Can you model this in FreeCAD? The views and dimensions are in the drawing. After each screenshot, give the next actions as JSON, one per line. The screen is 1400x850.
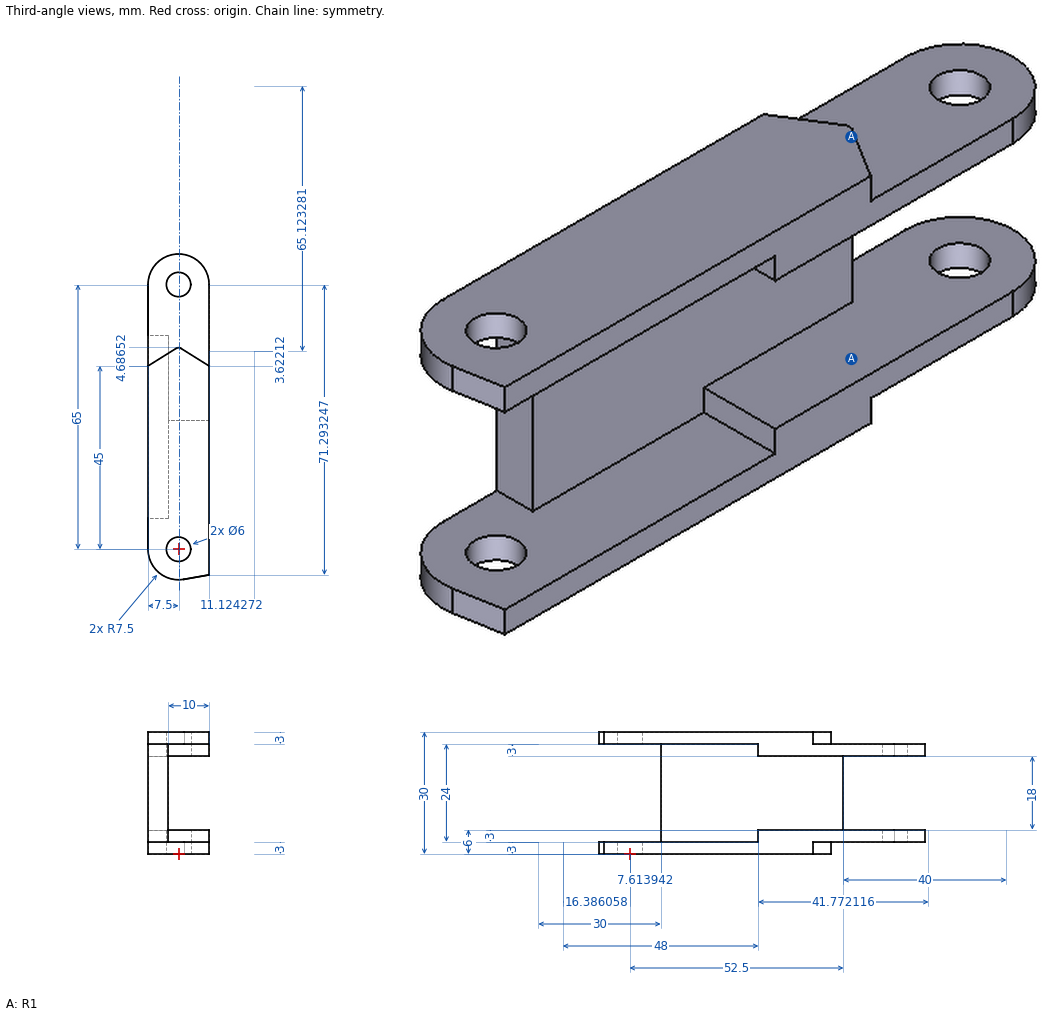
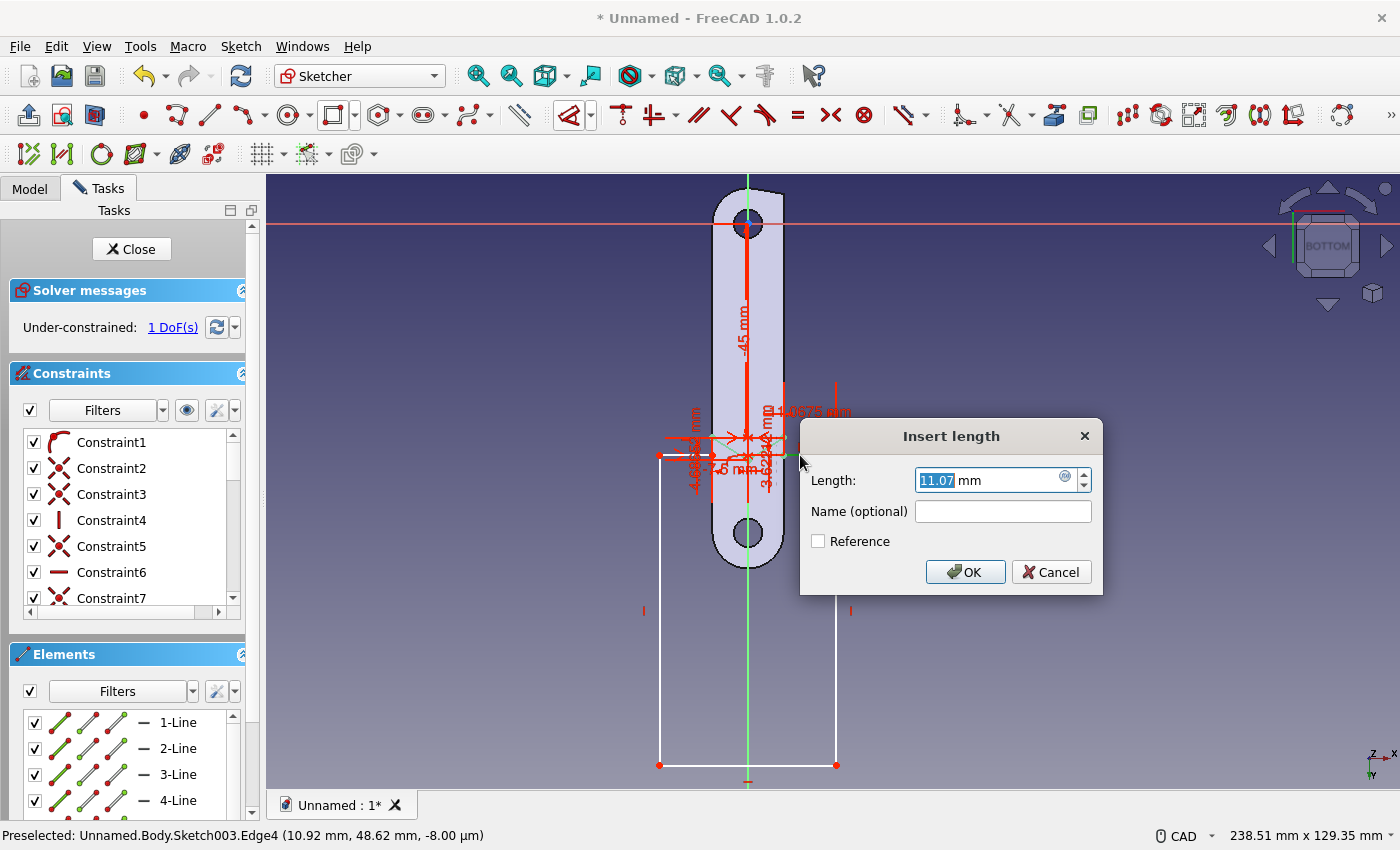
{"action": "type", "text": "11.124272"}
{"action": "key", "text": "Return"}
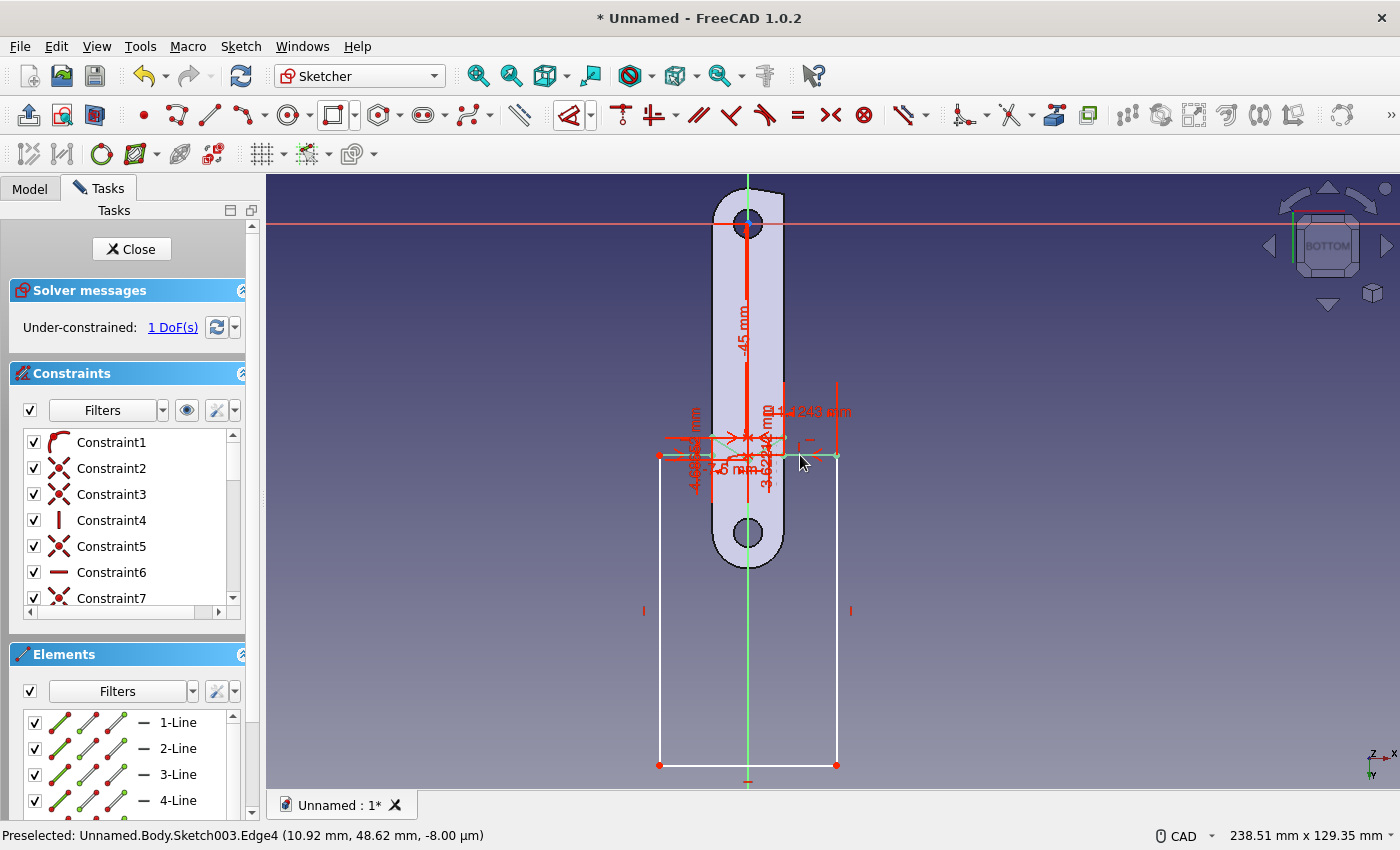
{"action": "left_click", "coordinate": [837, 548]}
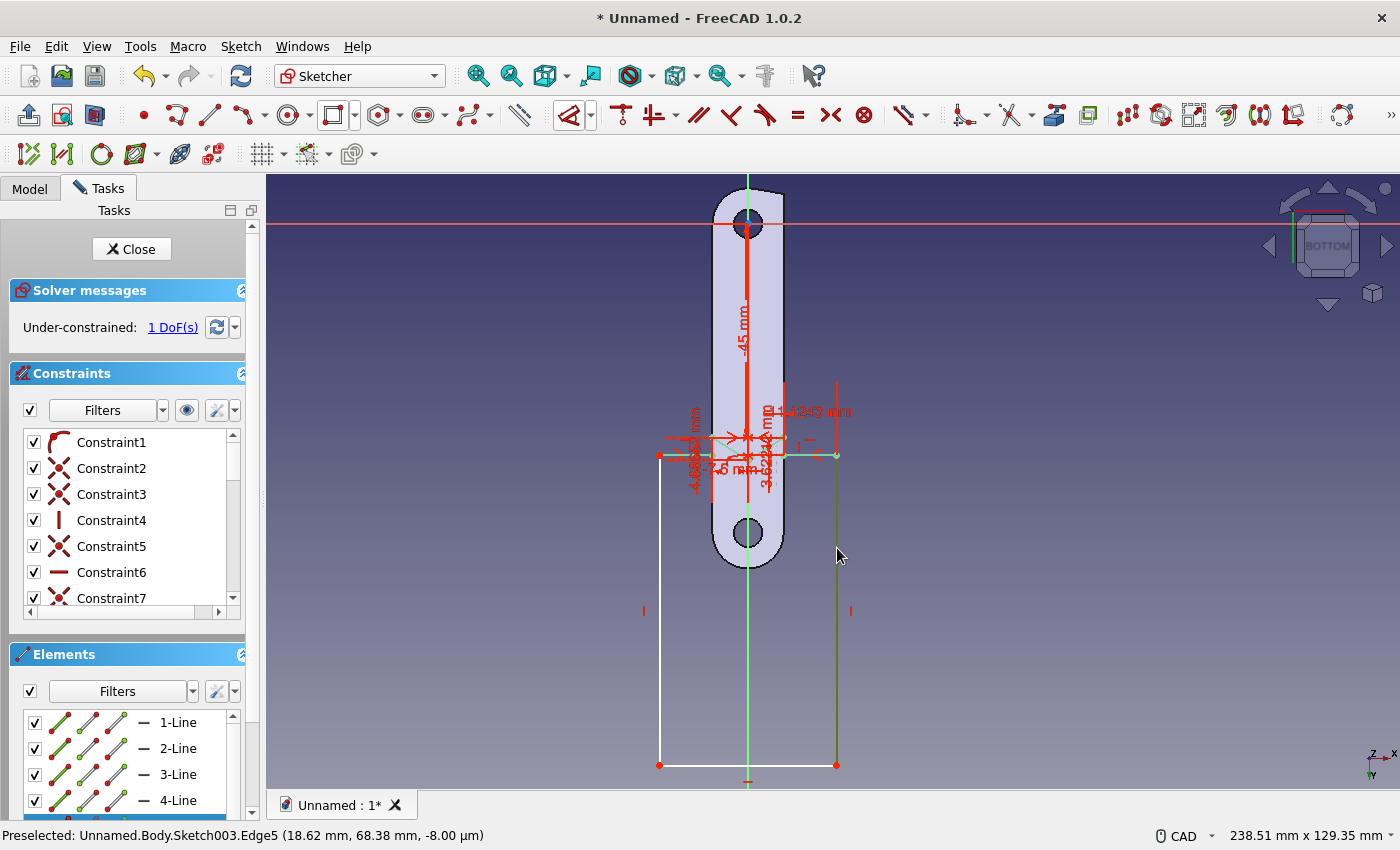
{"action": "key", "text": "i"}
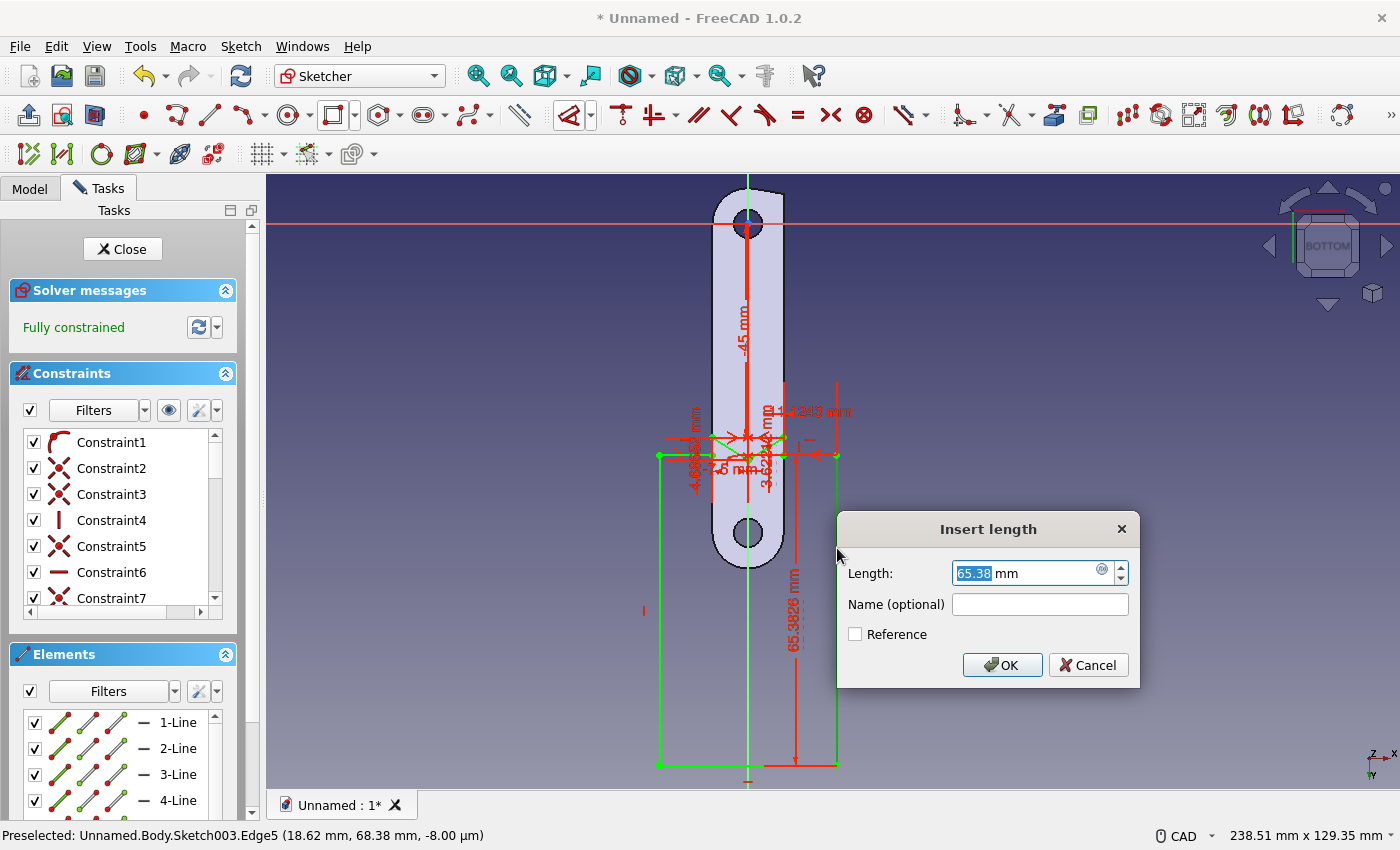
{"action": "type", "text": "65.123281"}
{"action": "key", "text": "Return"}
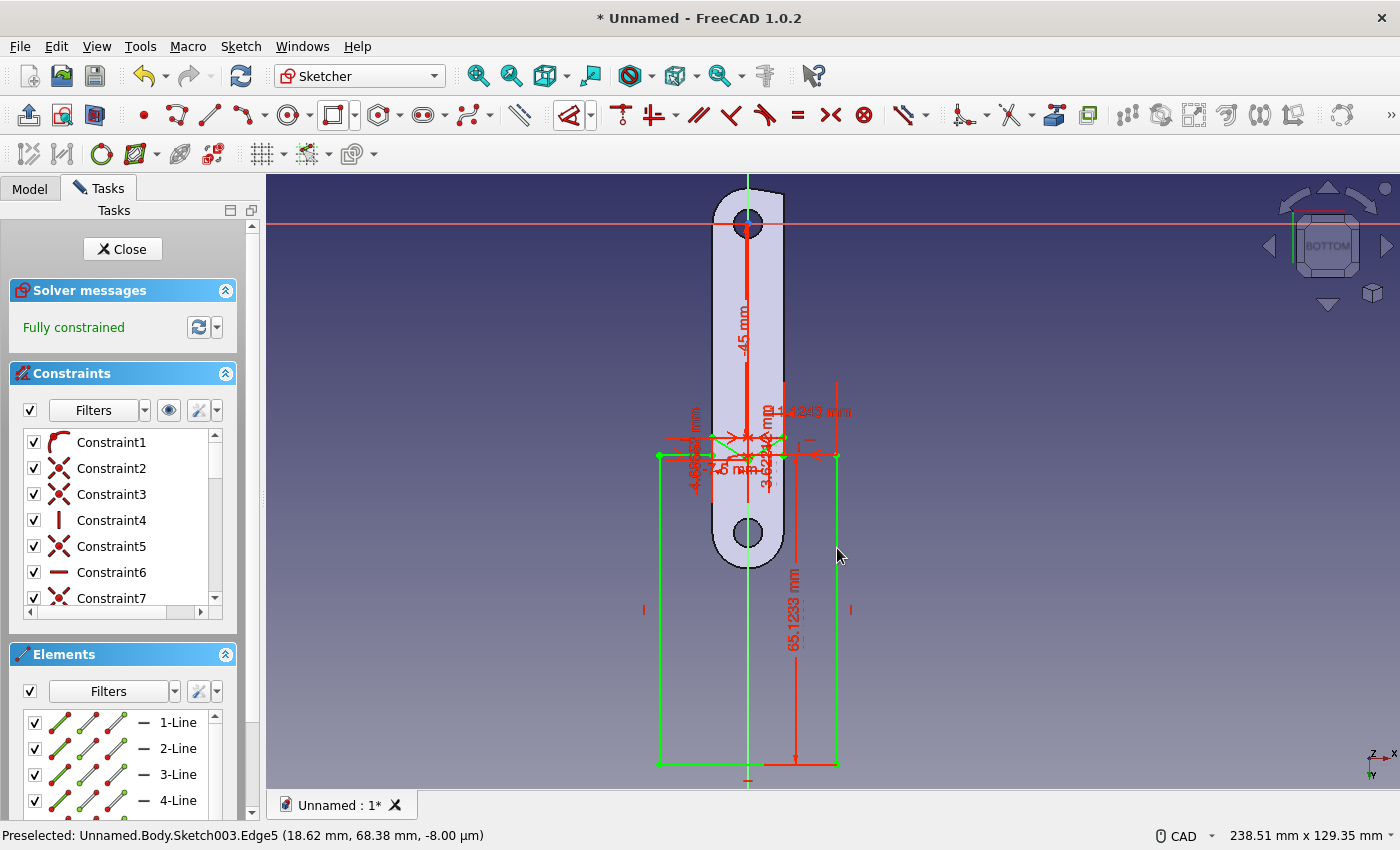
{"action": "left_click", "coordinate": [123, 249]}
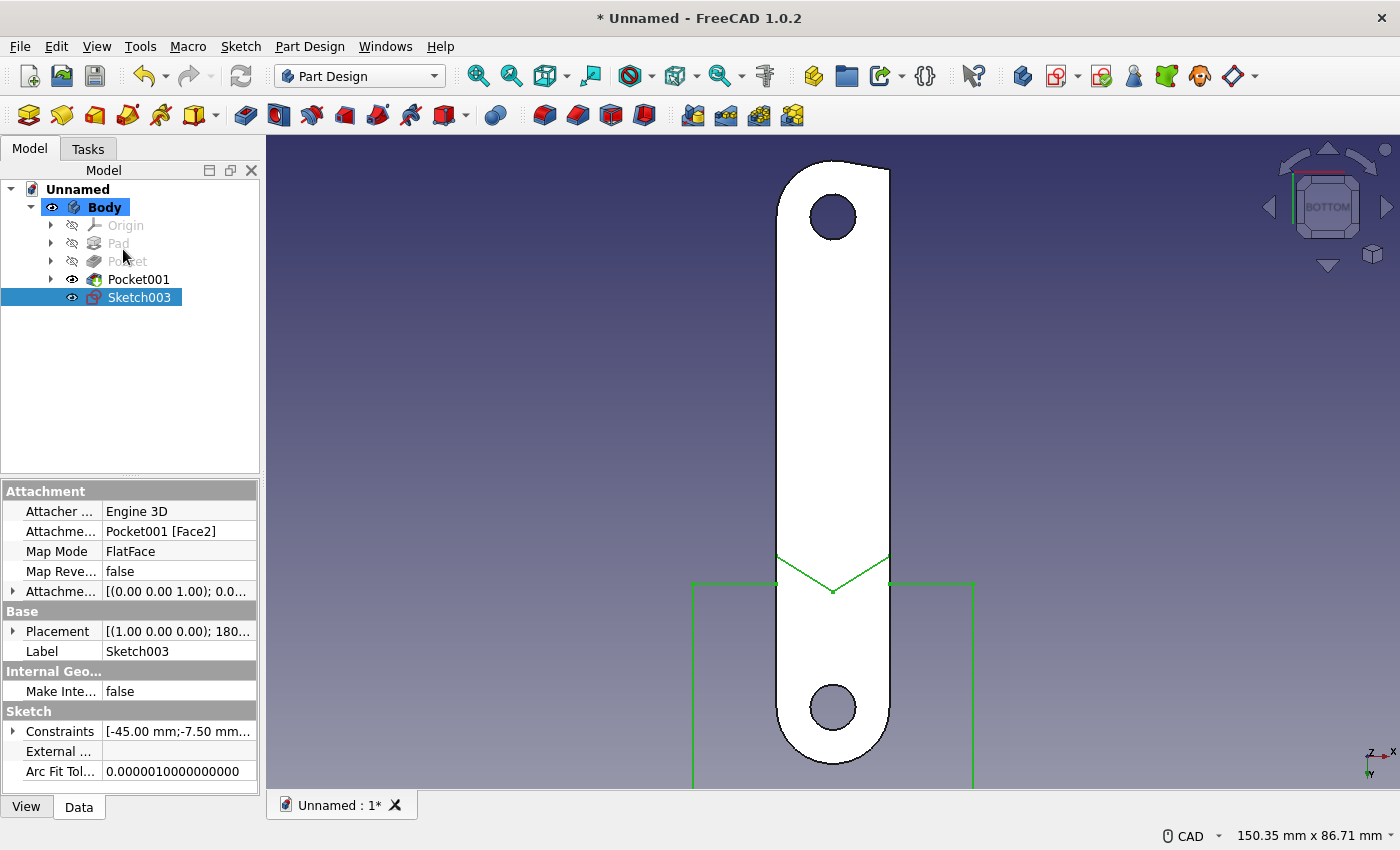
{"action": "left_click", "coordinate": [246, 116]}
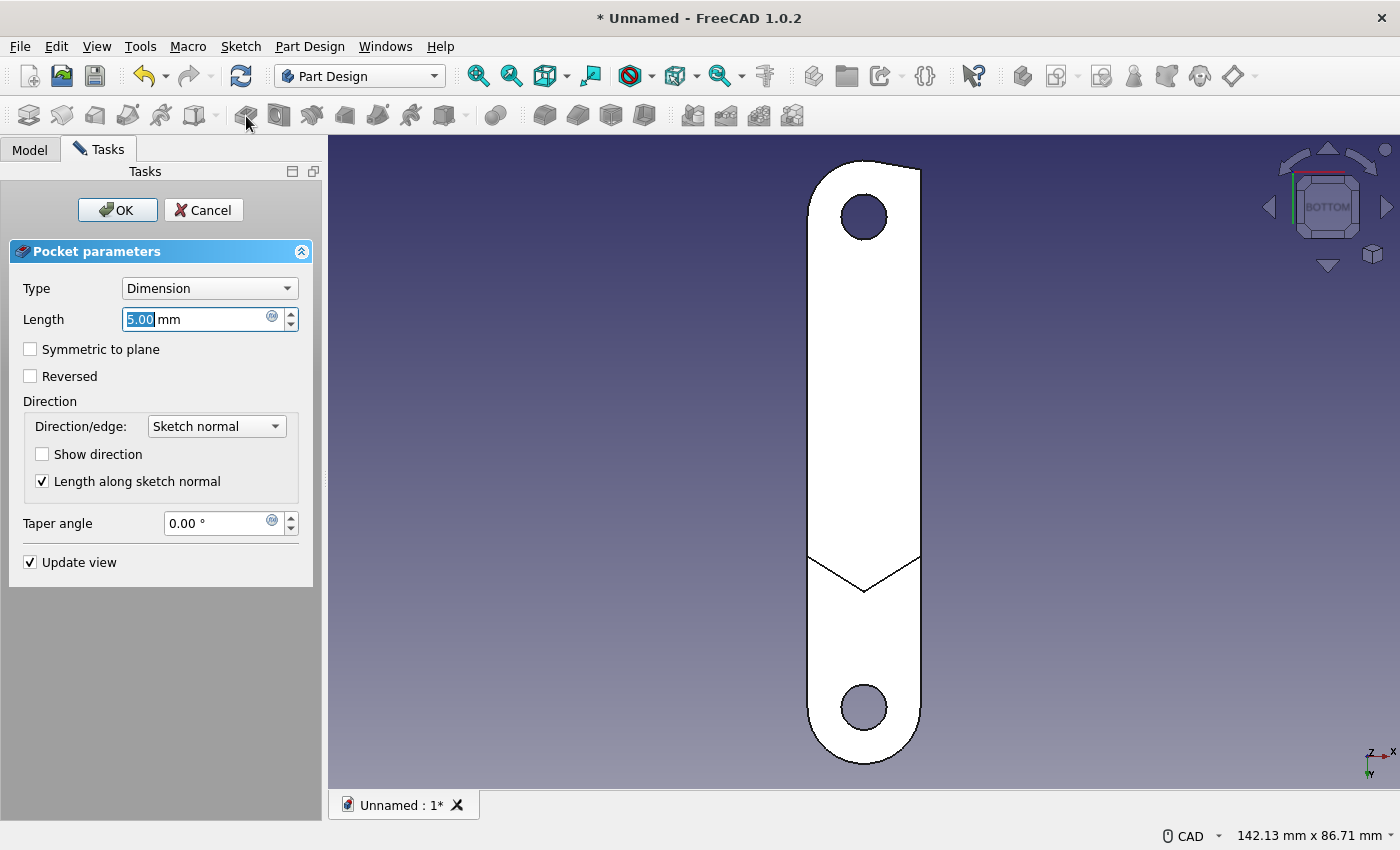
{"action": "type", "text": "3"}
{"action": "key", "text": "Tab"}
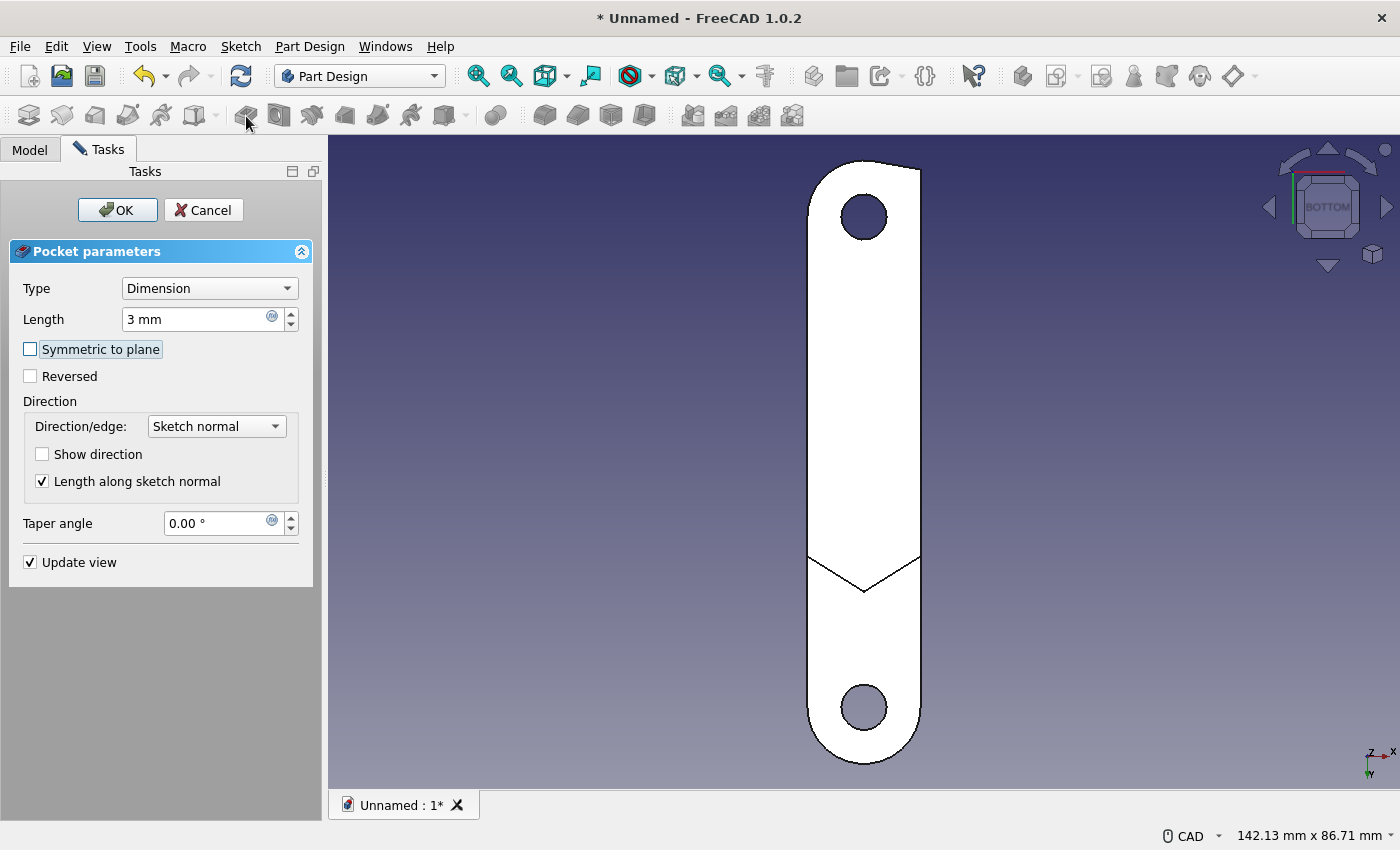
{"action": "left_click", "coordinate": [118, 210]}